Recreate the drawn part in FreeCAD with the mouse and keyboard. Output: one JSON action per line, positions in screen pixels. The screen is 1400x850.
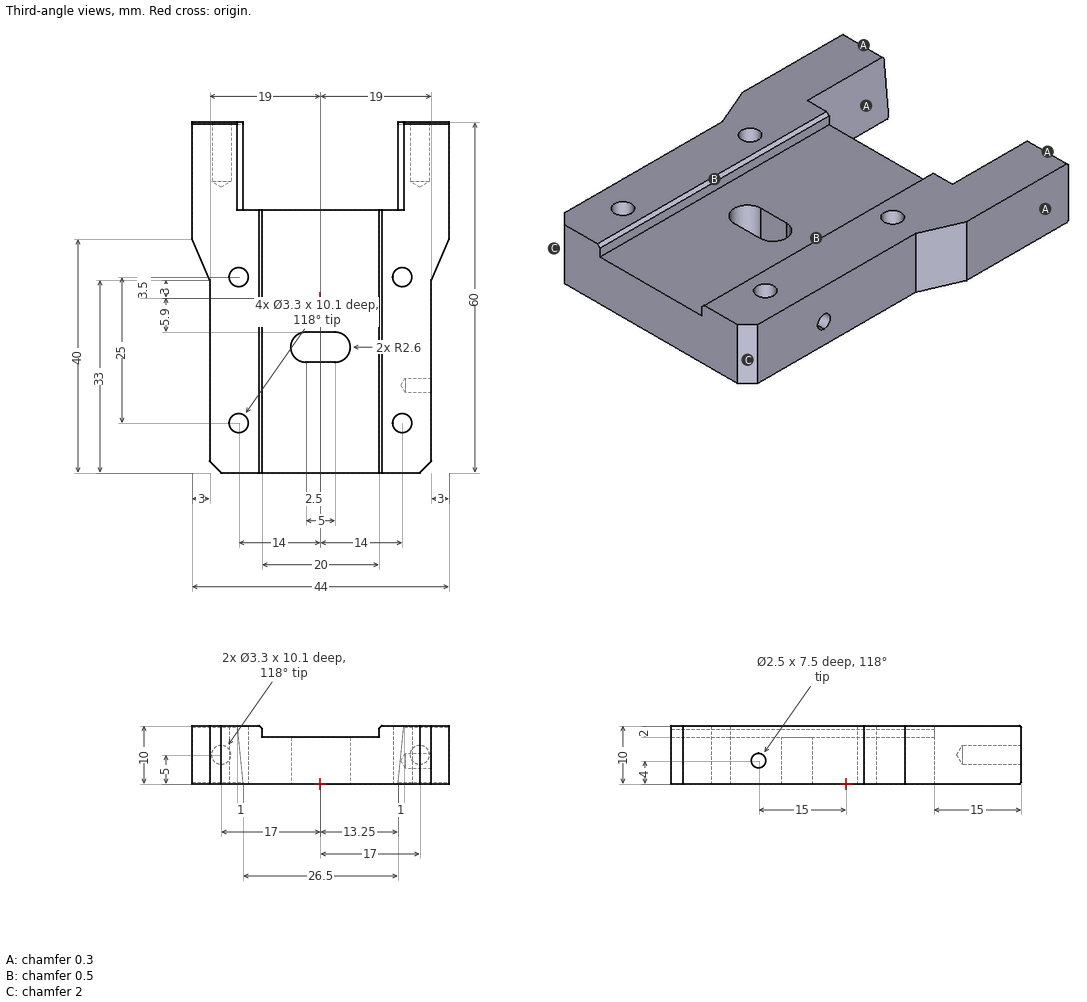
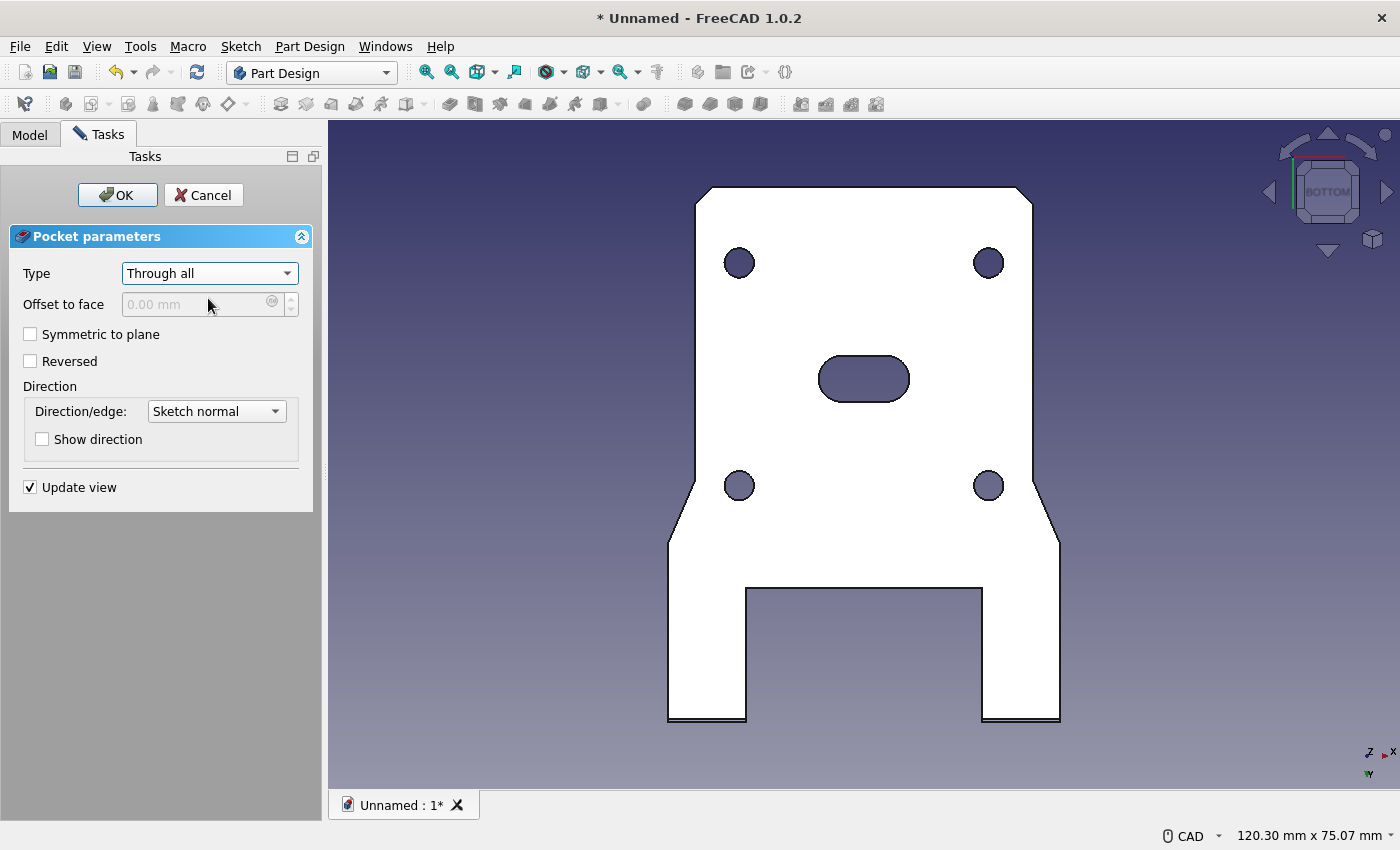
{"action": "left_click", "coordinate": [118, 195]}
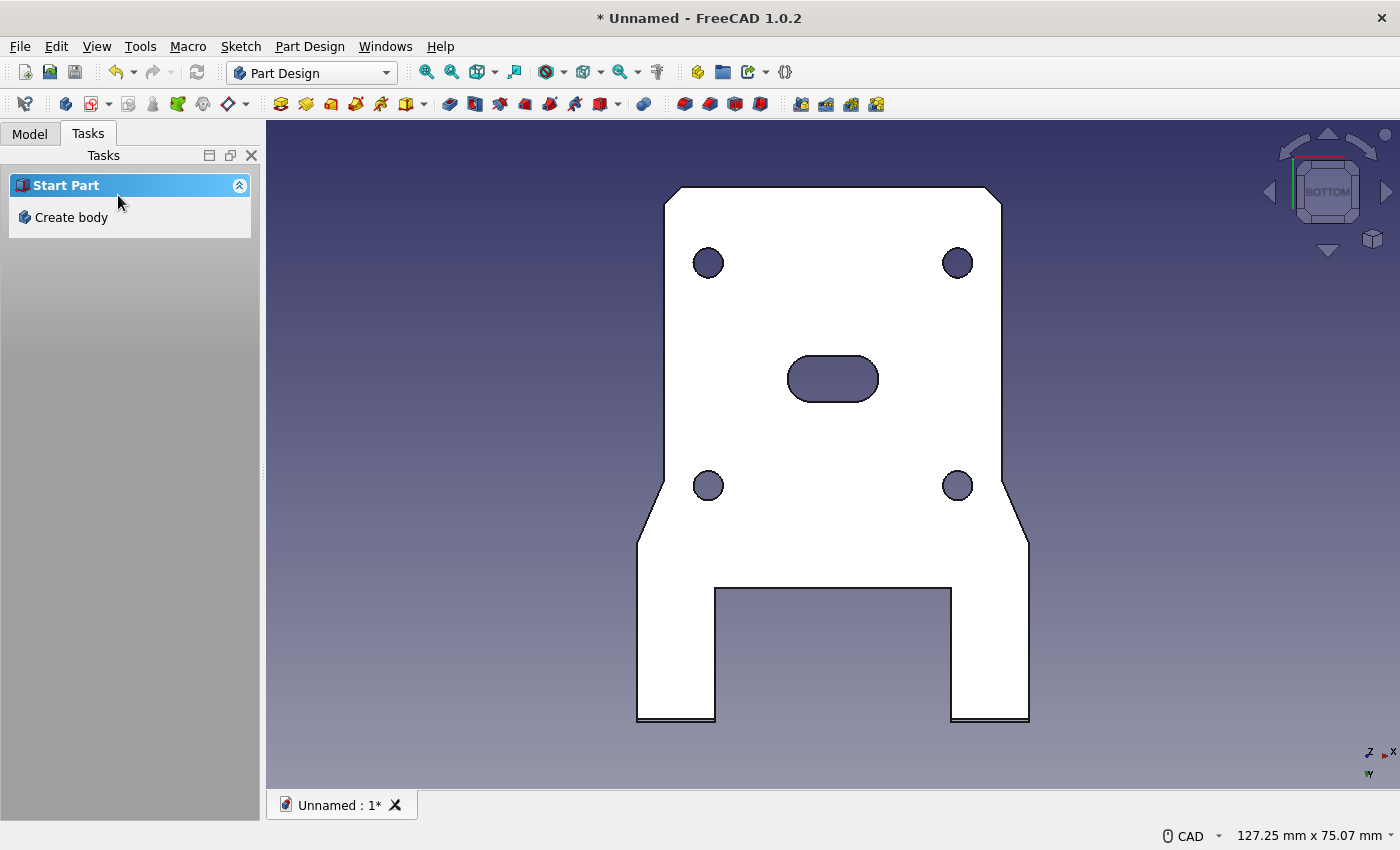
{"action": "key", "text": "0"}